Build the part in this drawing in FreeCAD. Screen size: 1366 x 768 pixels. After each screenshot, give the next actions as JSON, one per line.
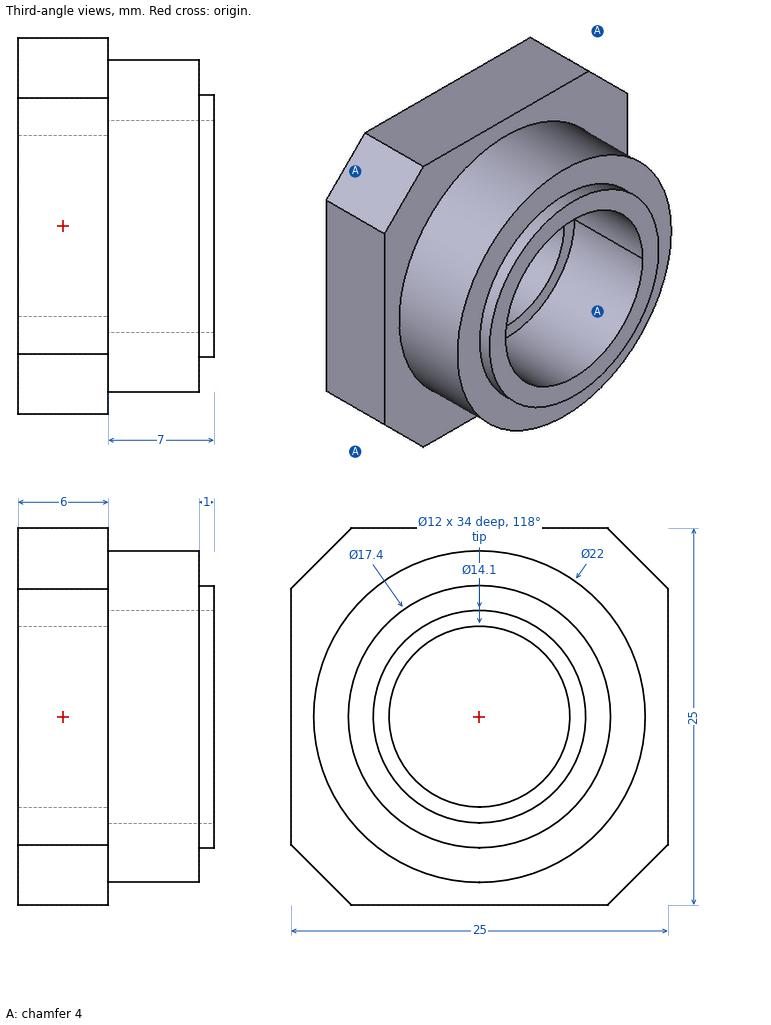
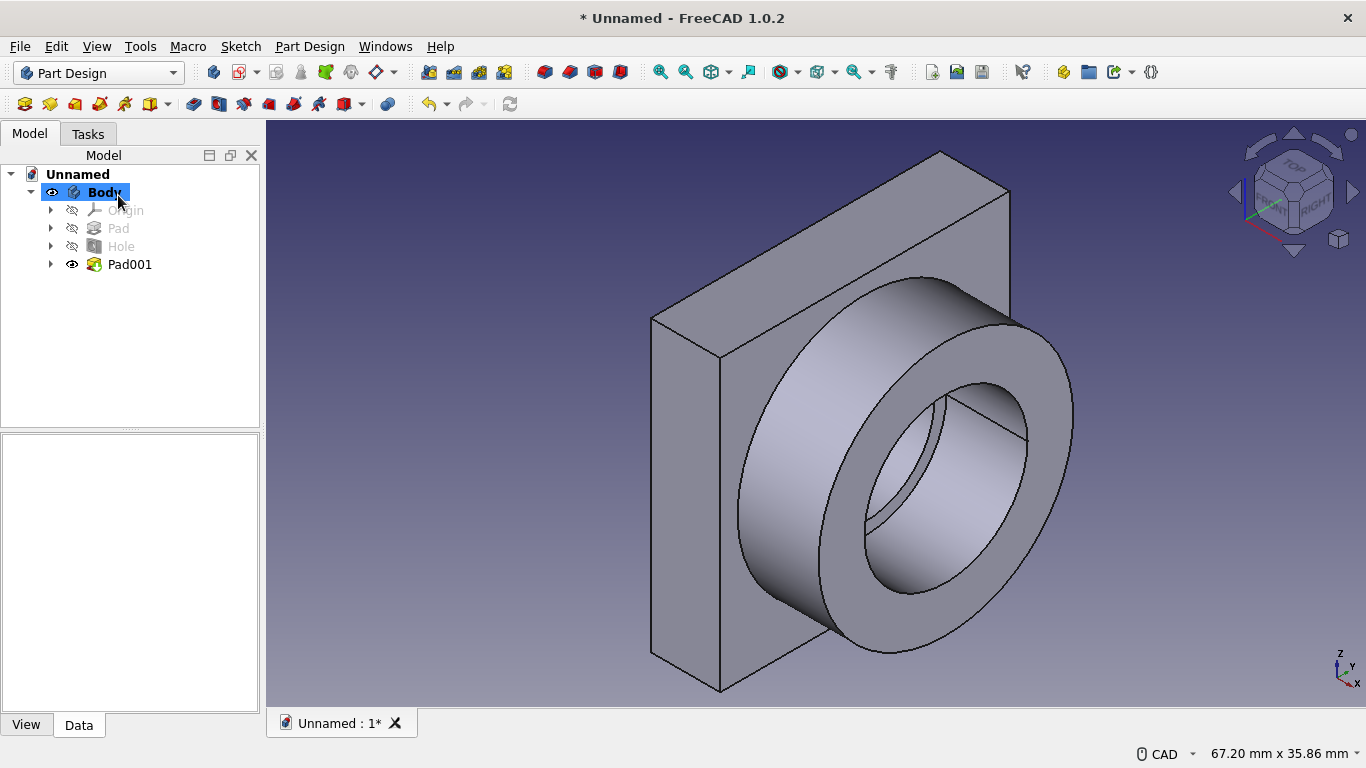
{"action": "left_click", "coordinate": [661, 72]}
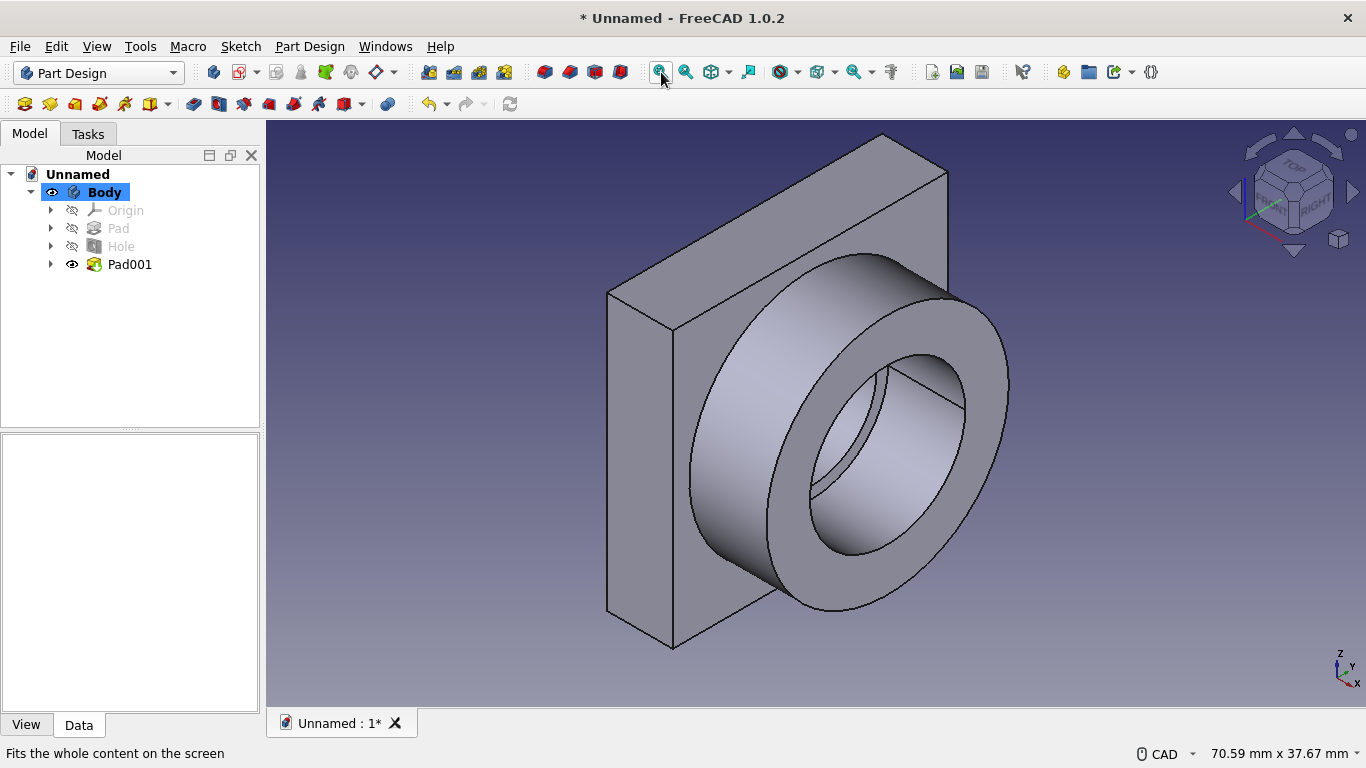
{"action": "left_click", "coordinate": [51, 210]}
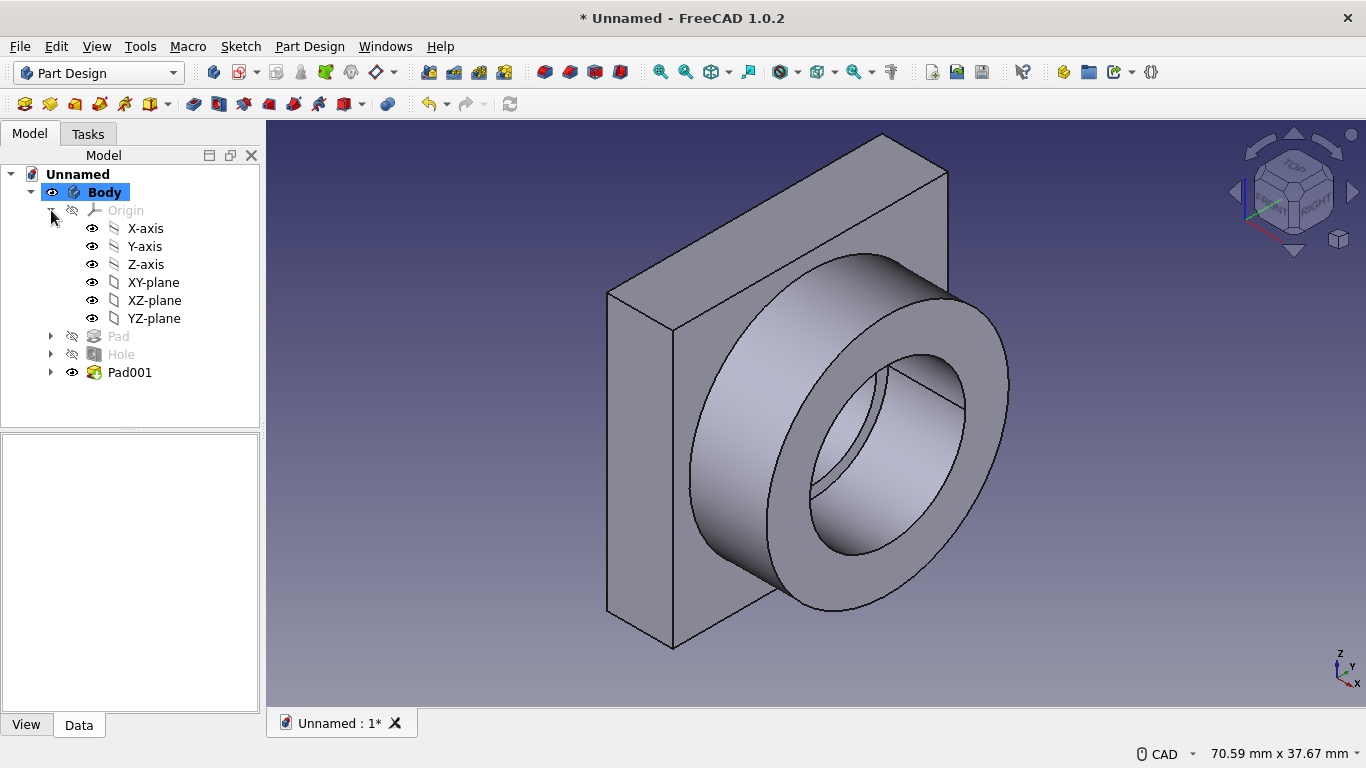
{"action": "left_click", "coordinate": [137, 318]}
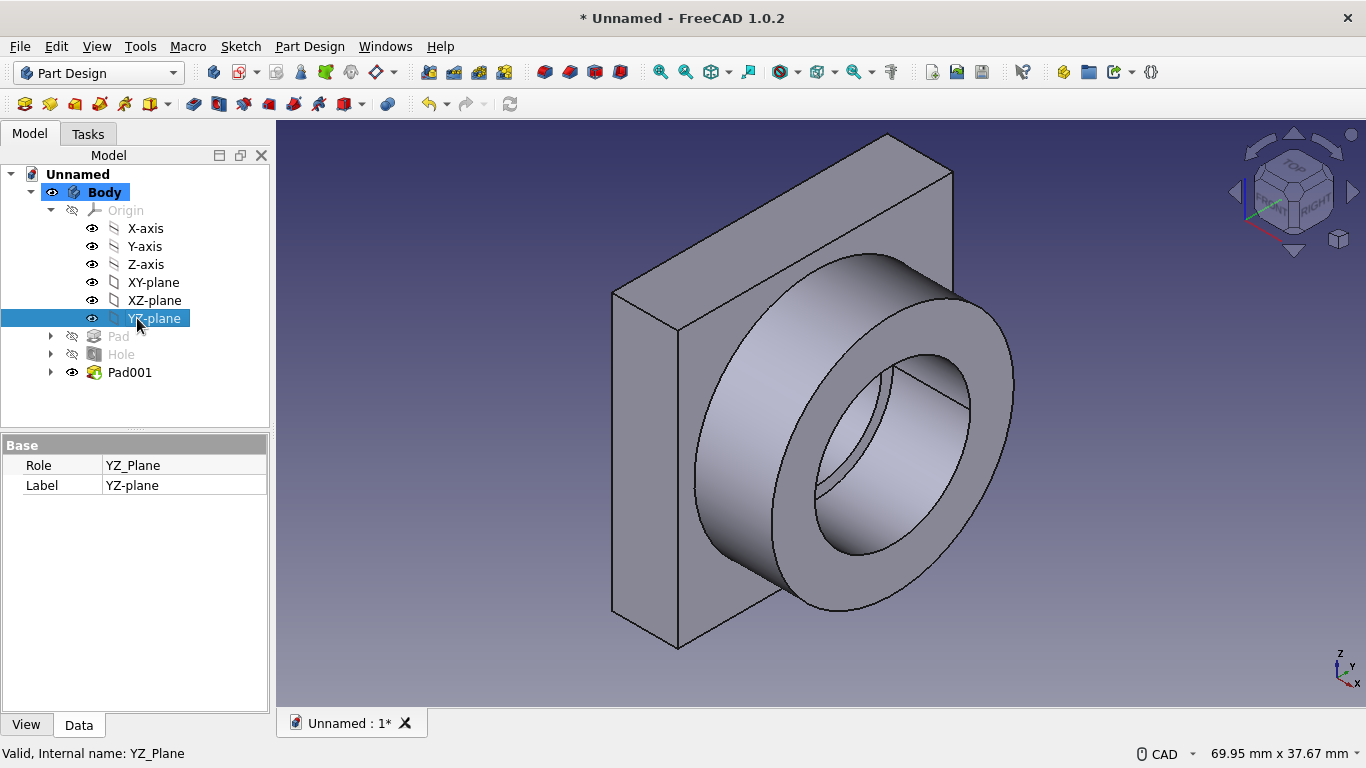
{"action": "left_click", "coordinate": [376, 72]}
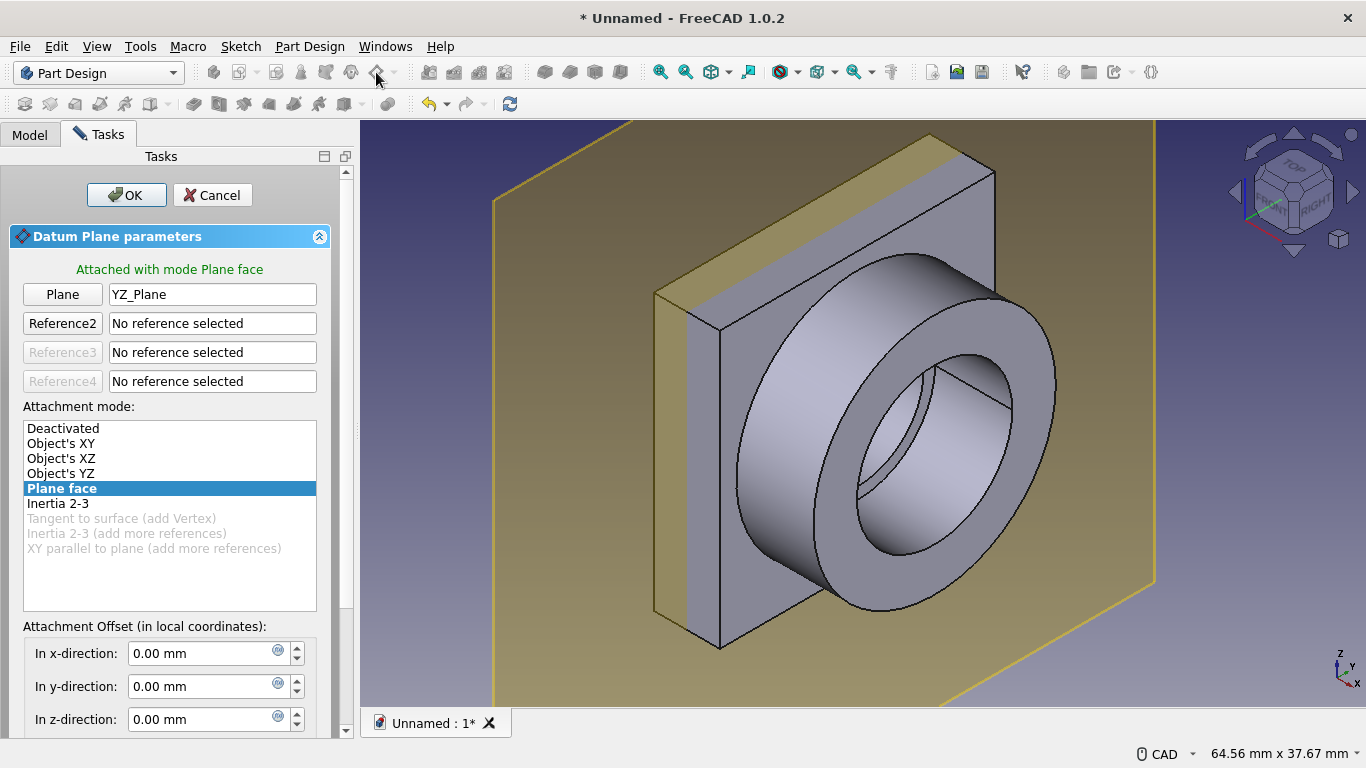
{"action": "triple_click", "coordinate": [210, 720]}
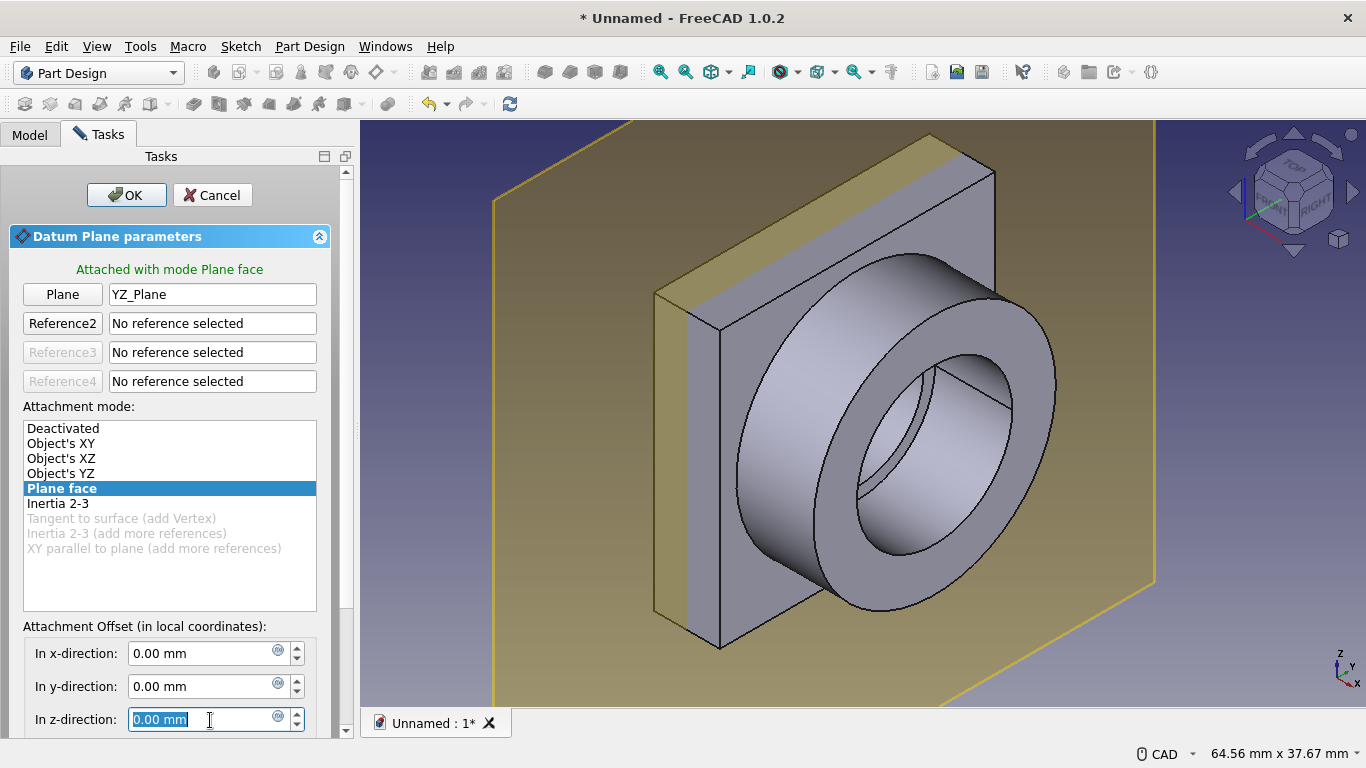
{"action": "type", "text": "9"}
{"action": "key", "text": "Tab"}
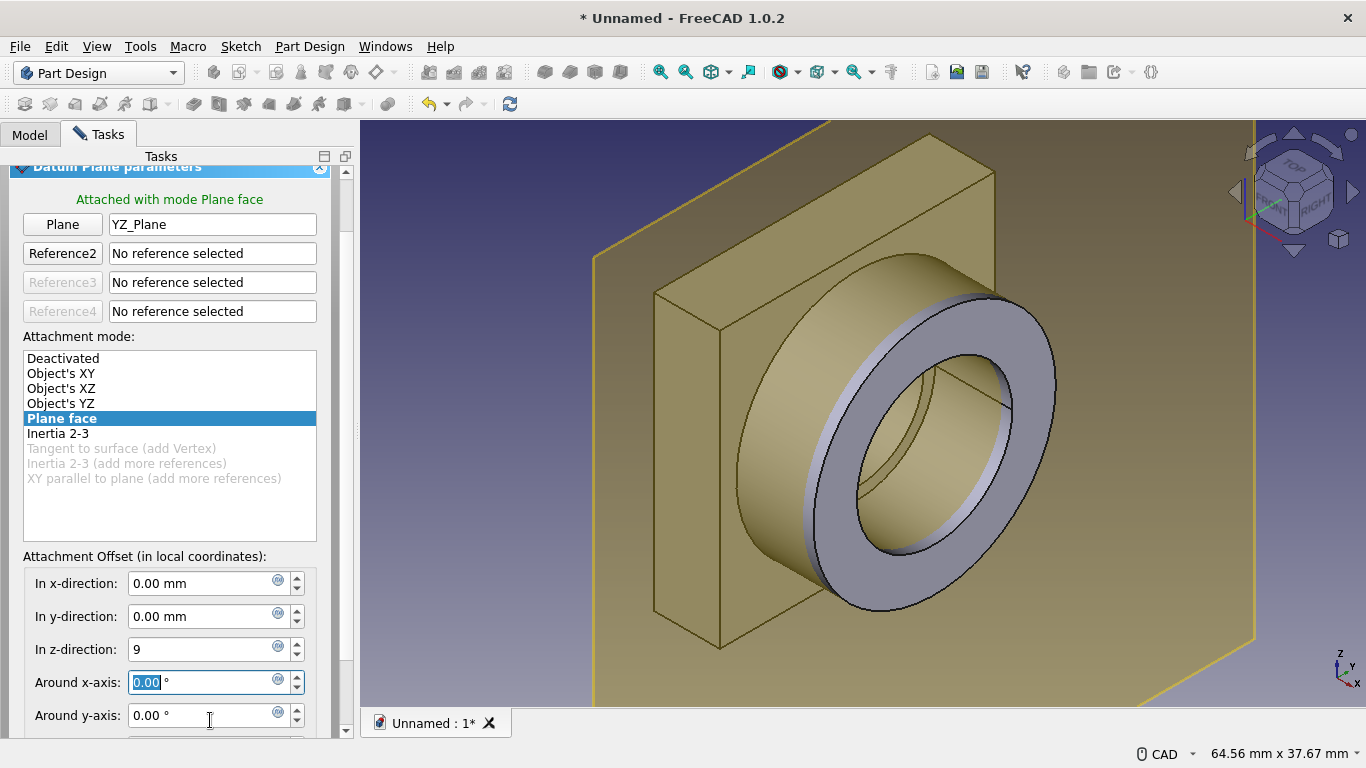
{"action": "scroll", "coordinate": [346, 452], "scroll_direction": "up", "scroll_amount": 2}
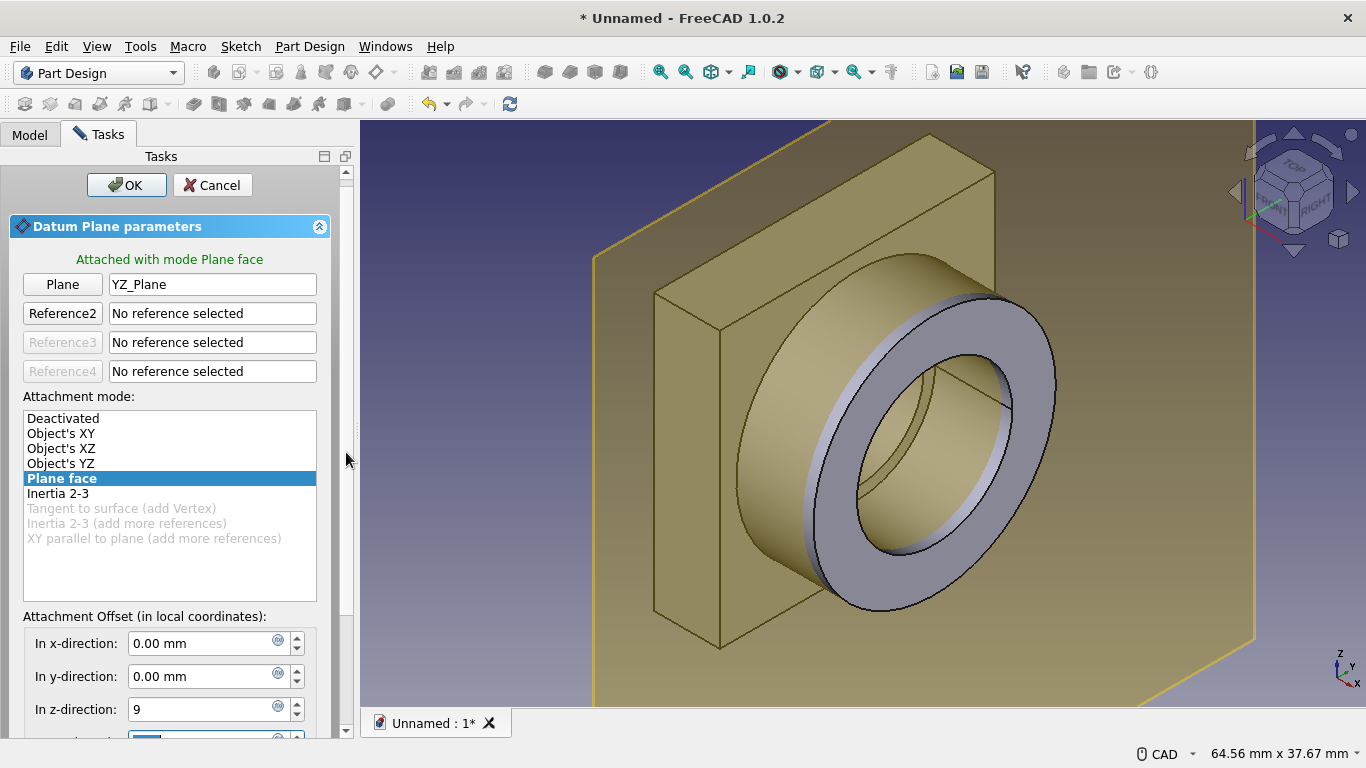
{"action": "left_click", "coordinate": [127, 195]}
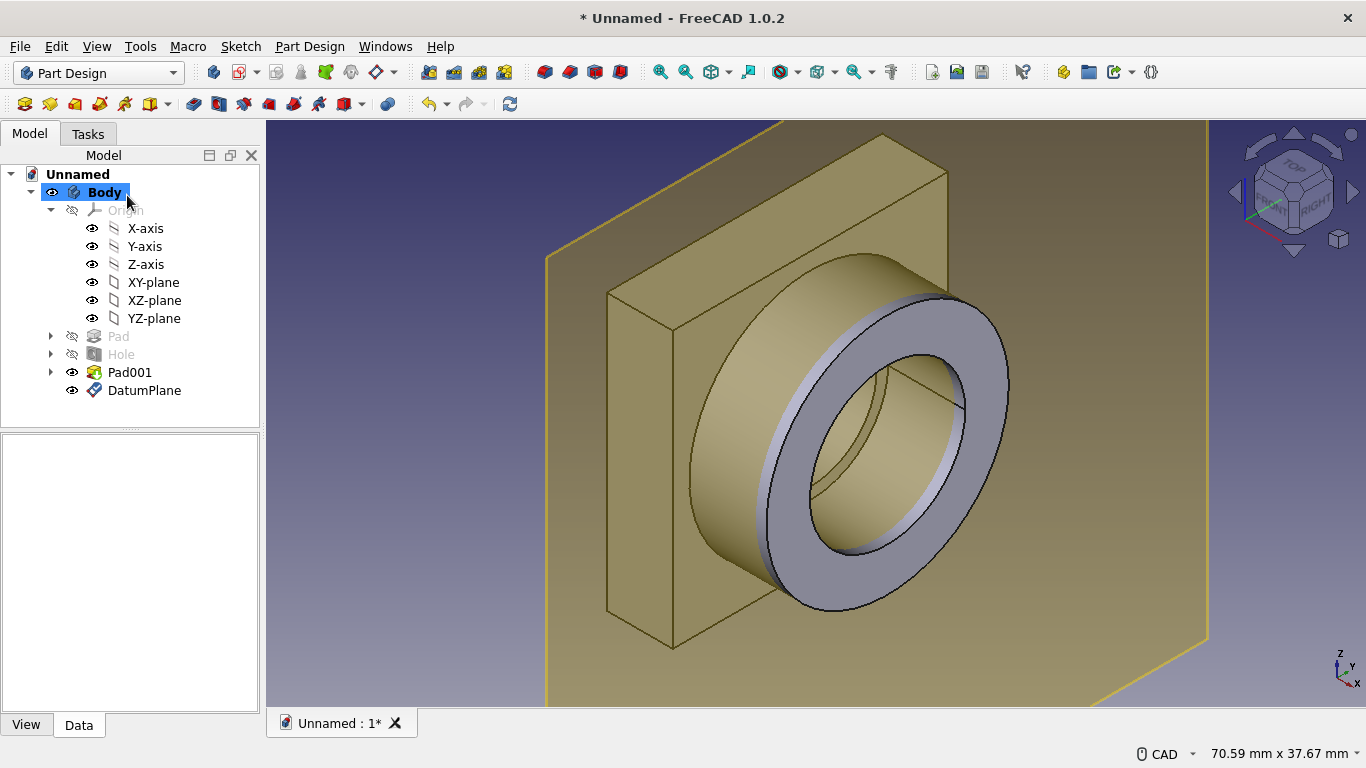
{"action": "left_click", "coordinate": [117, 390]}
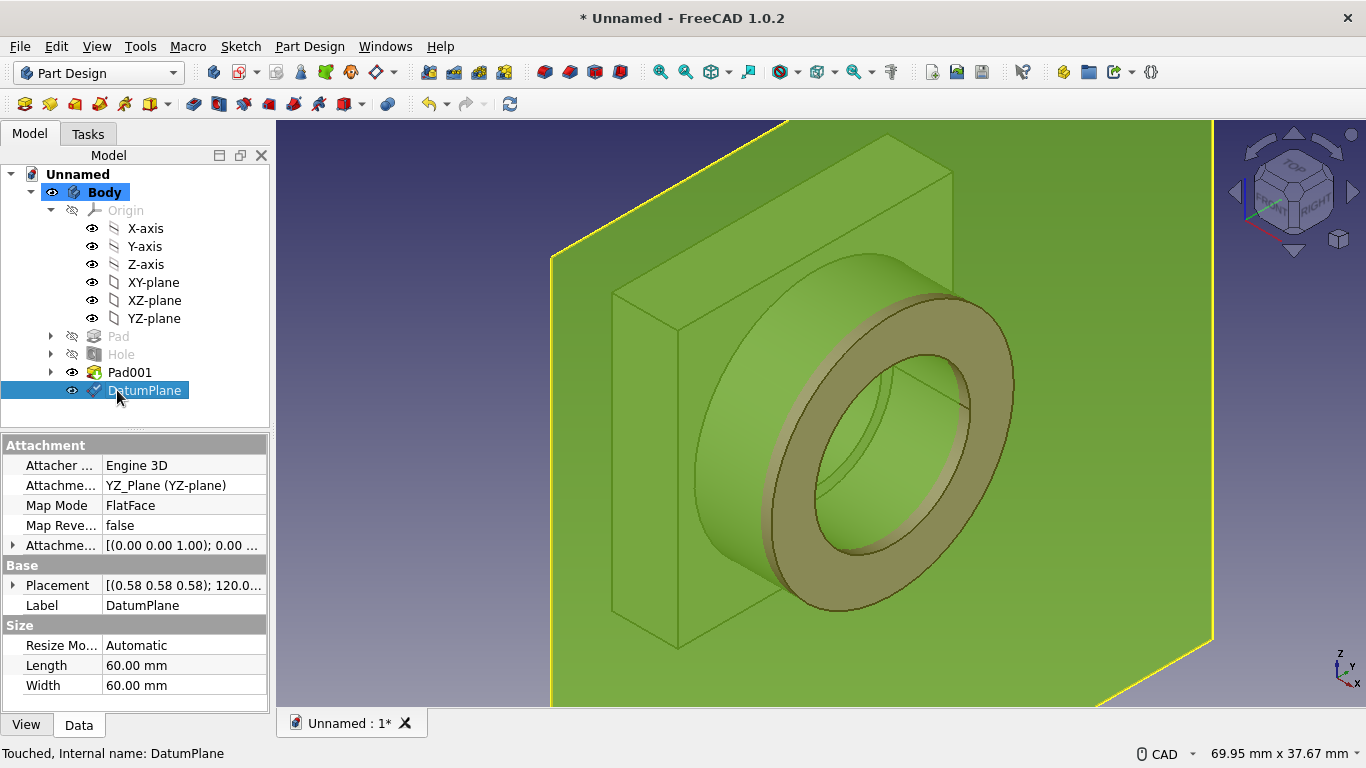
{"action": "left_click", "coordinate": [238, 72]}